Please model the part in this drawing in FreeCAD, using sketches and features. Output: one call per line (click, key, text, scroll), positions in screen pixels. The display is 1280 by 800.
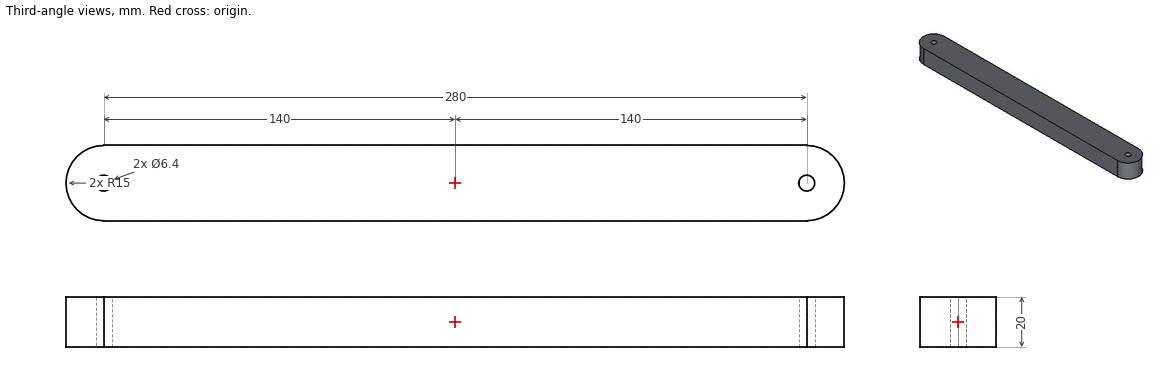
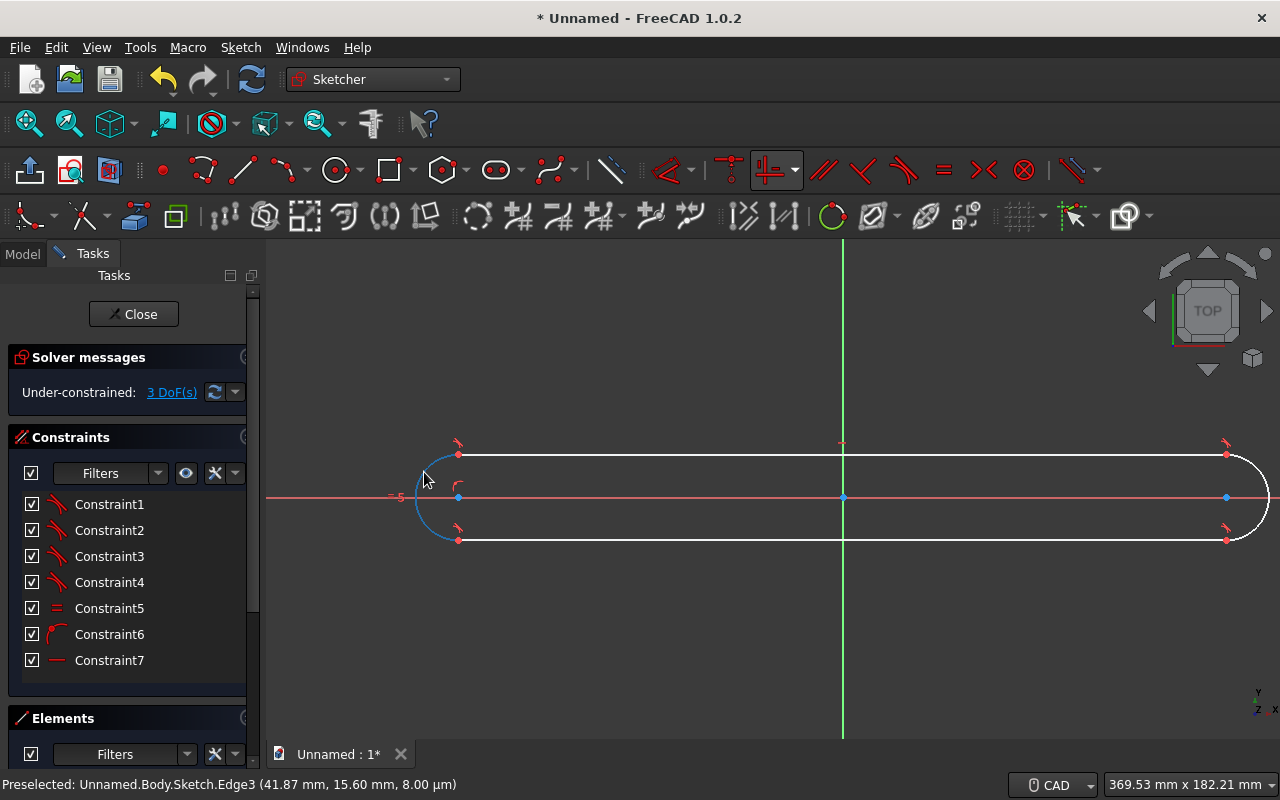
click(424, 472)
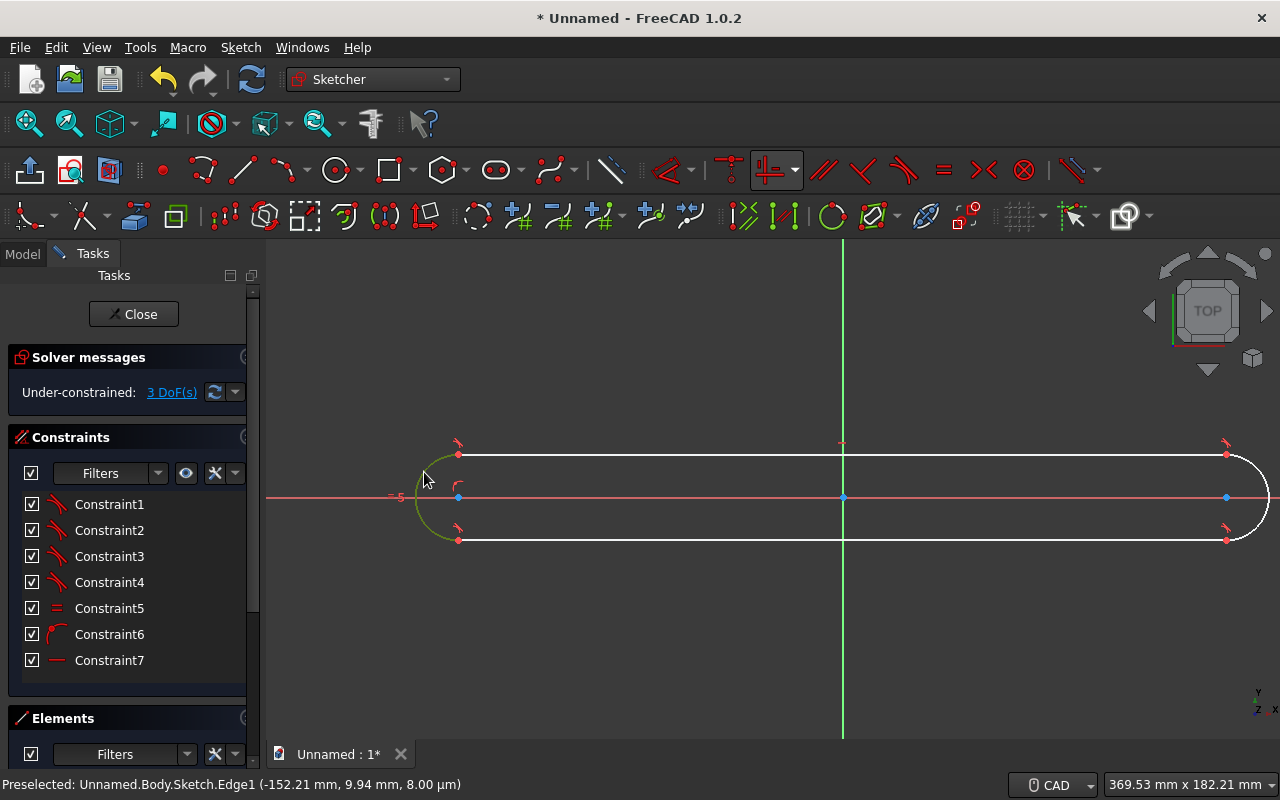
key(k)
key(r)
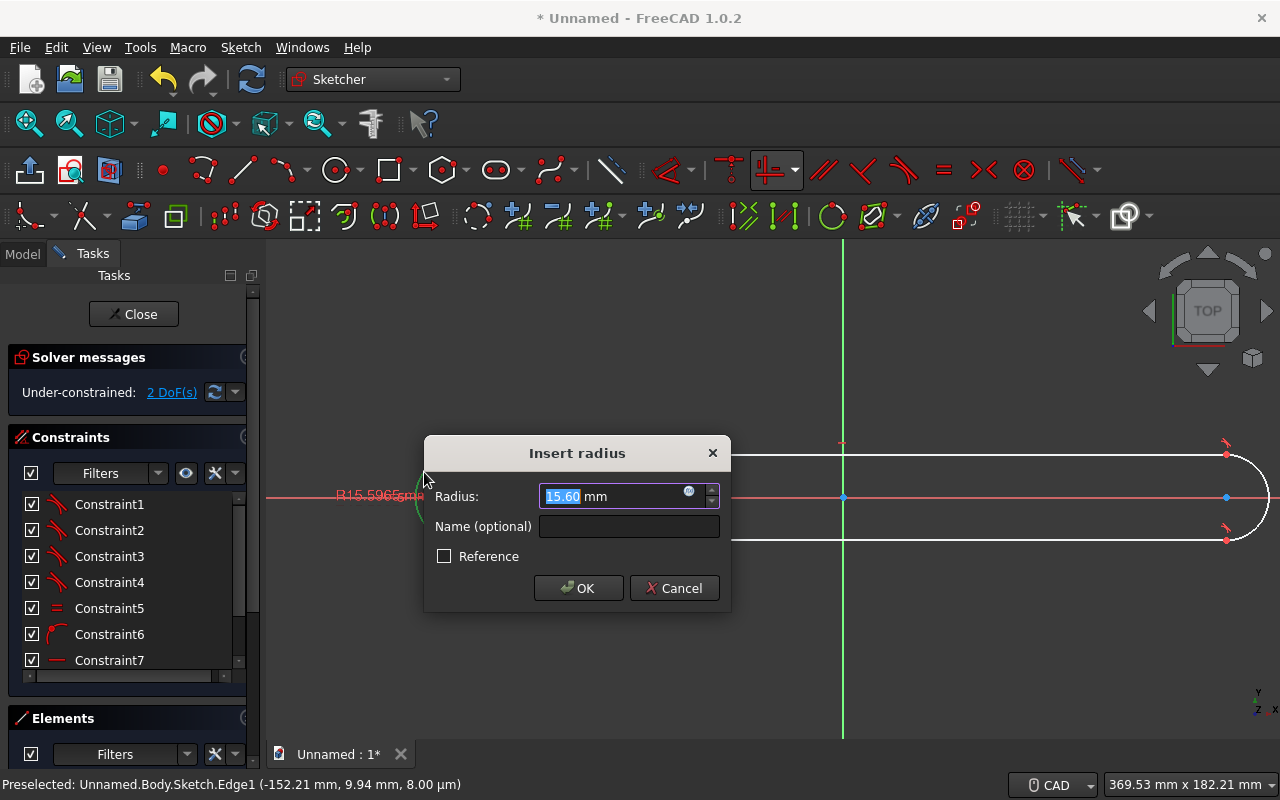
text(15)
key(Return)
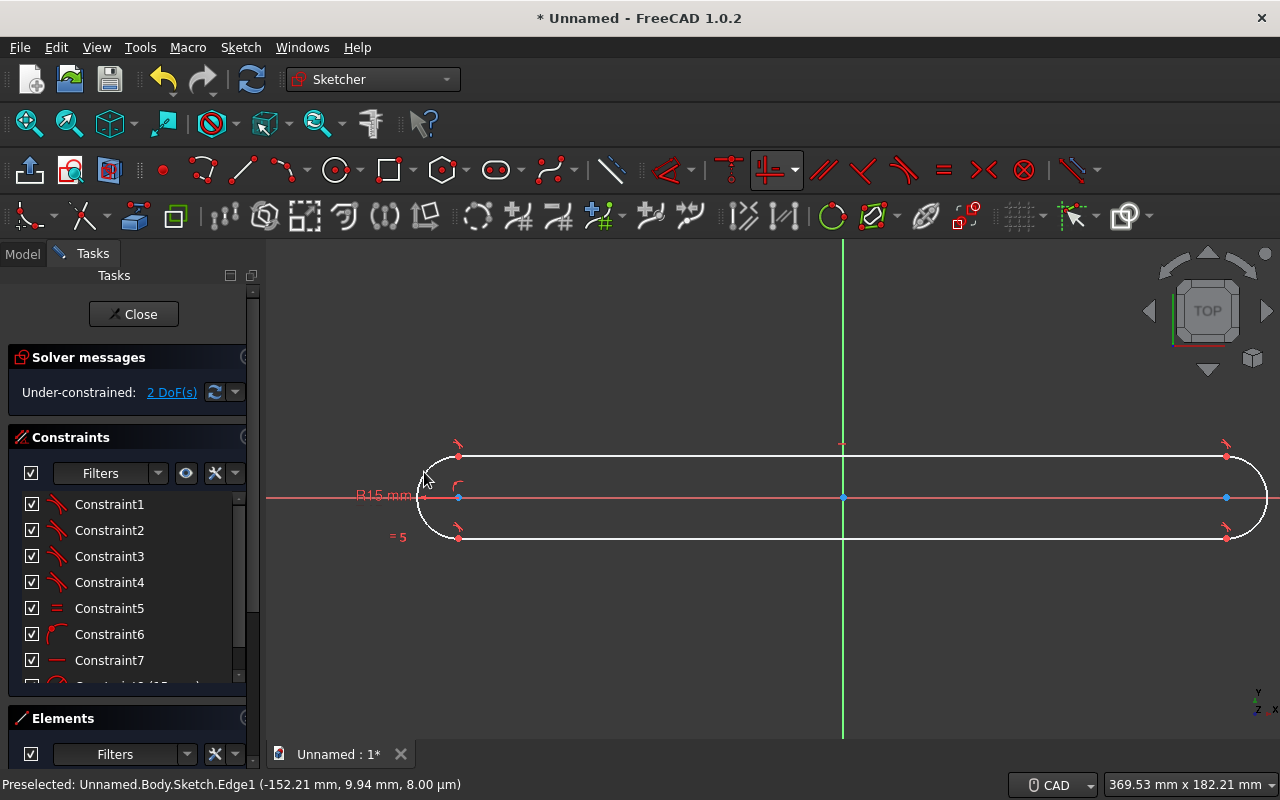
click(689, 456)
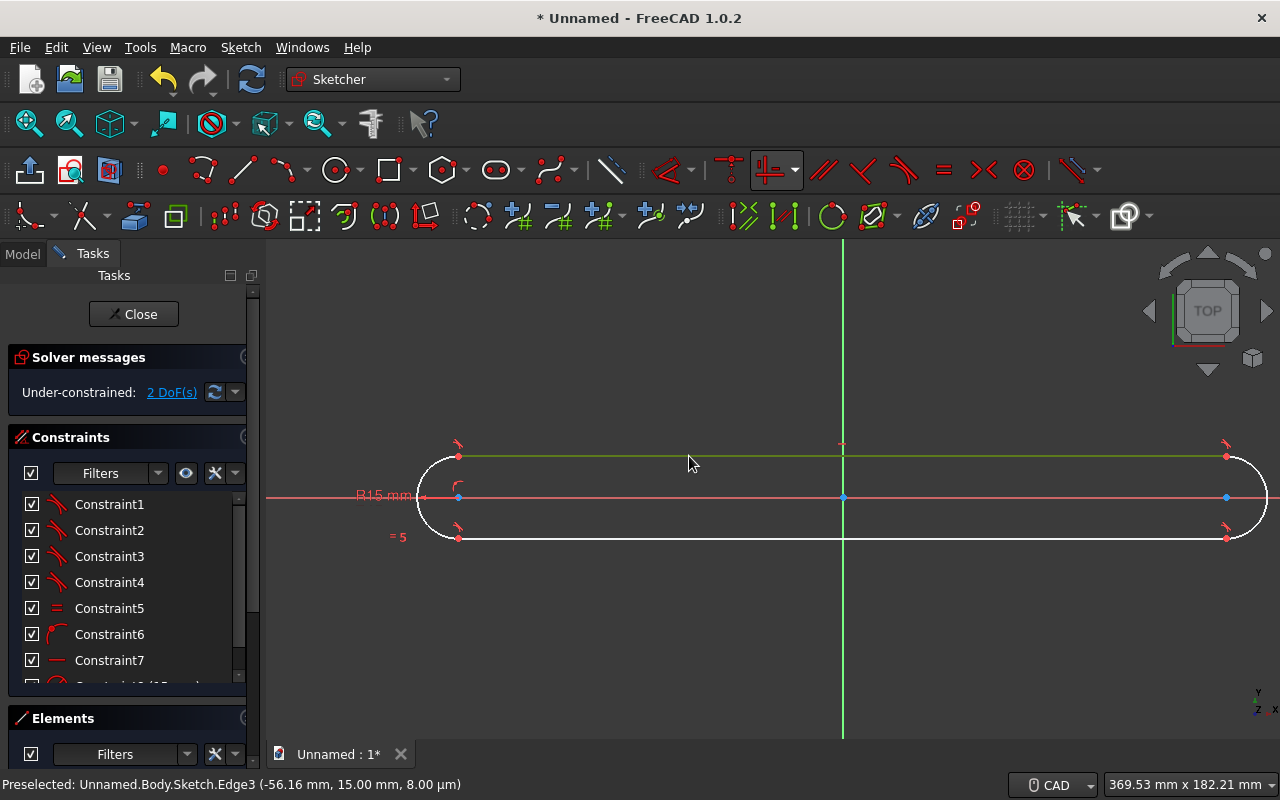
key(l)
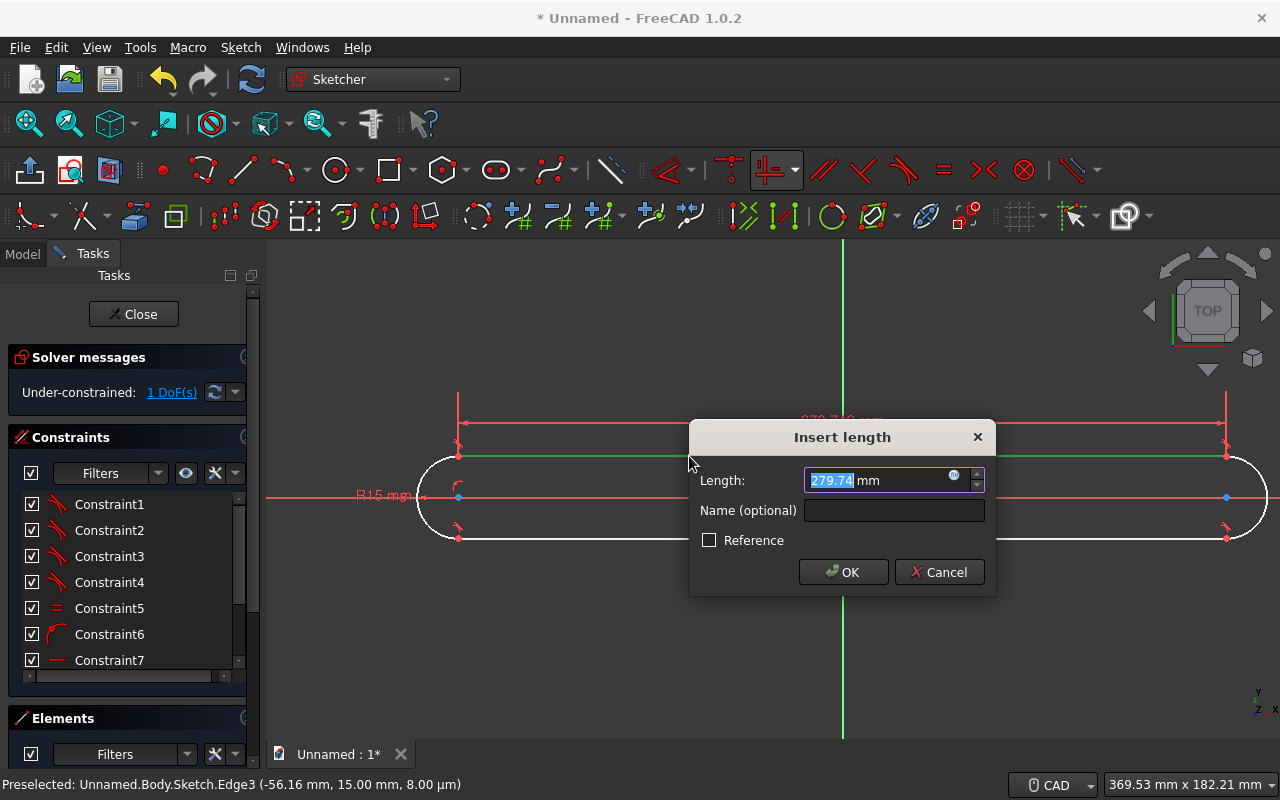
text(280)
key(Return)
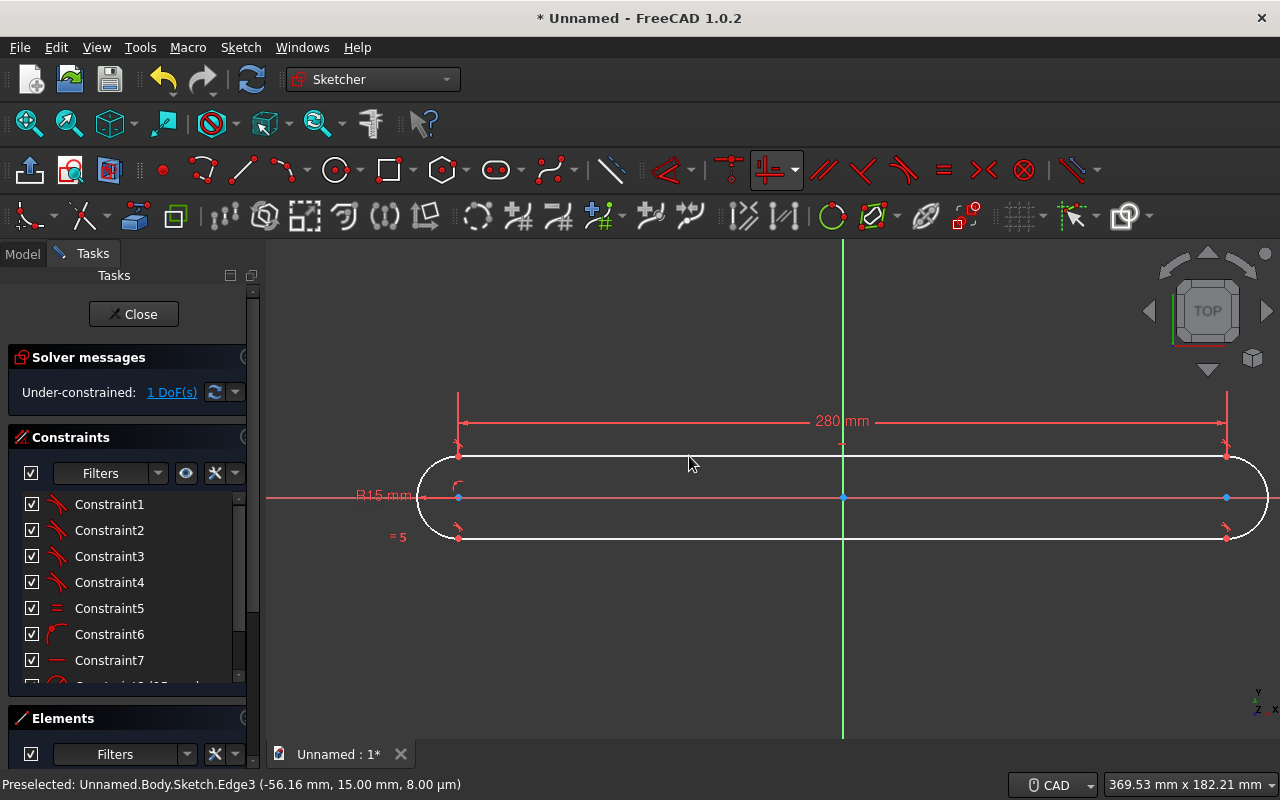
click(458, 456)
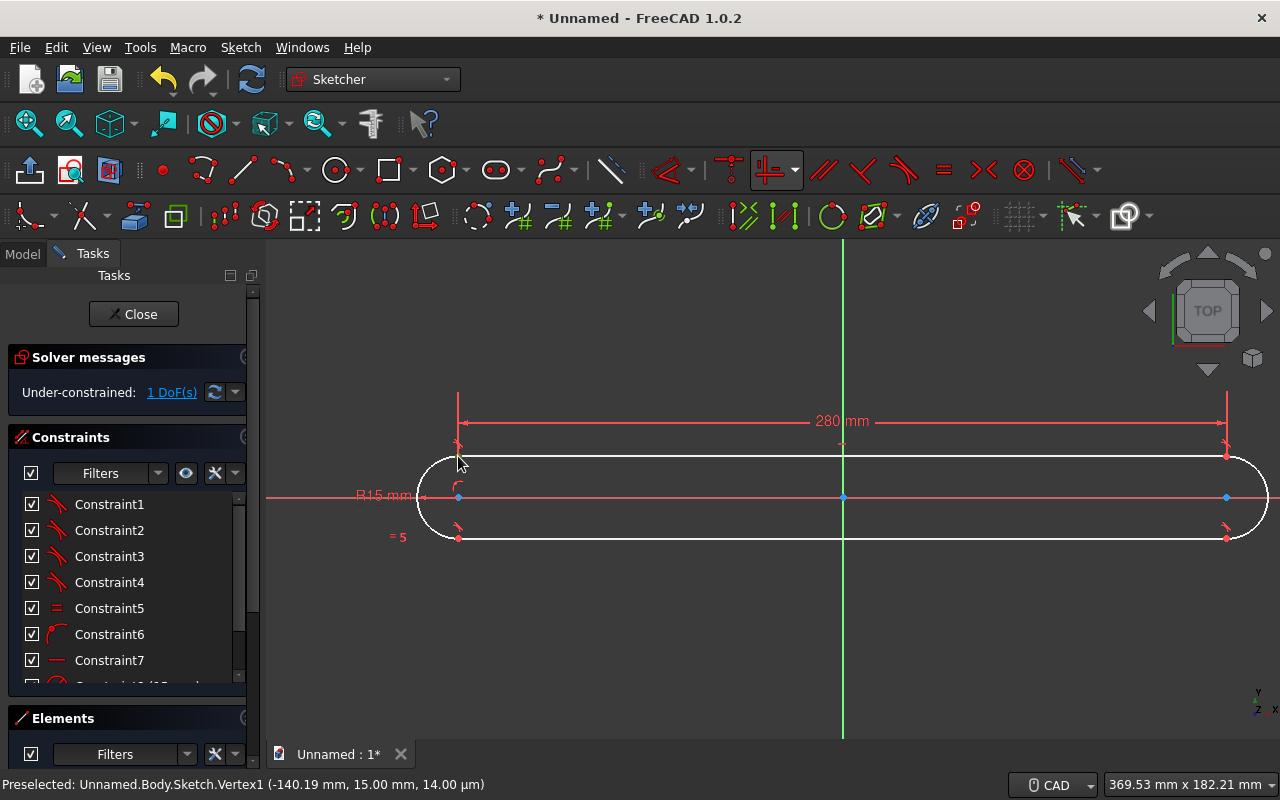
key(l)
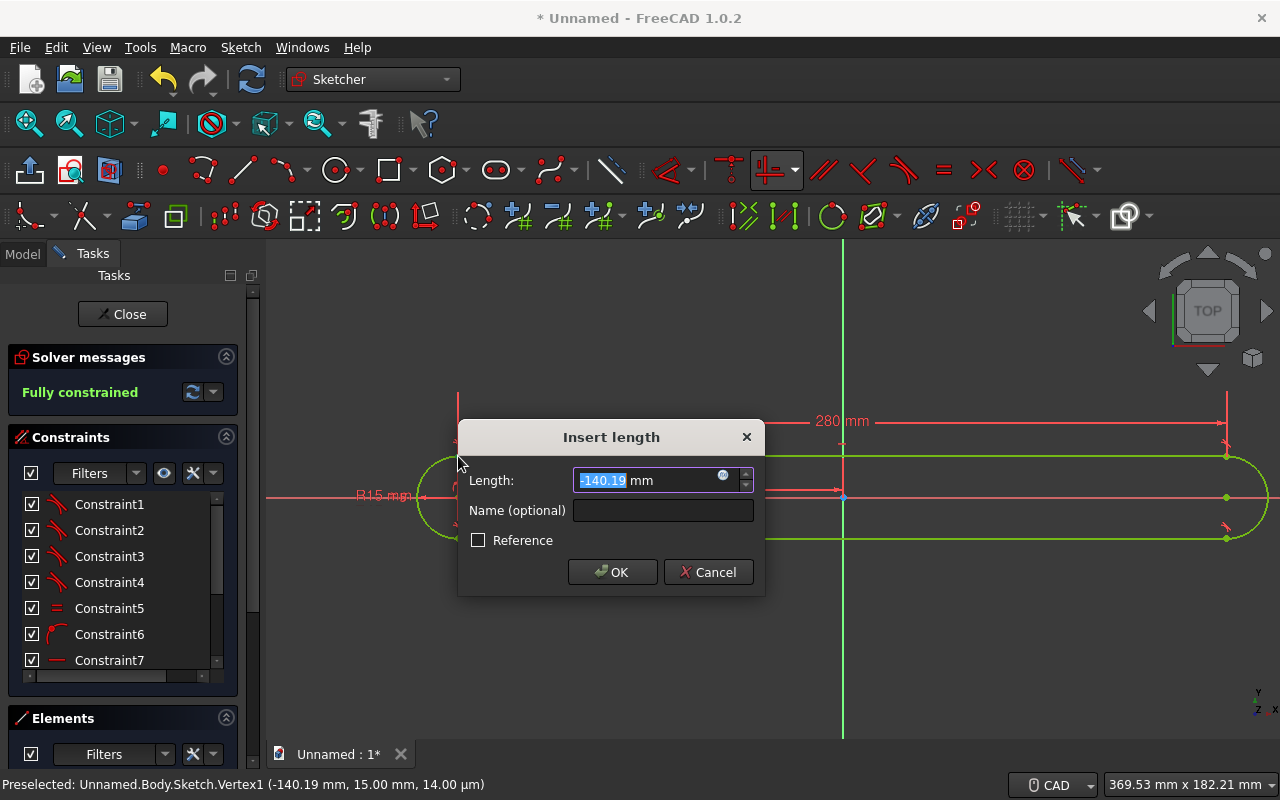
text(-140)
key(Return)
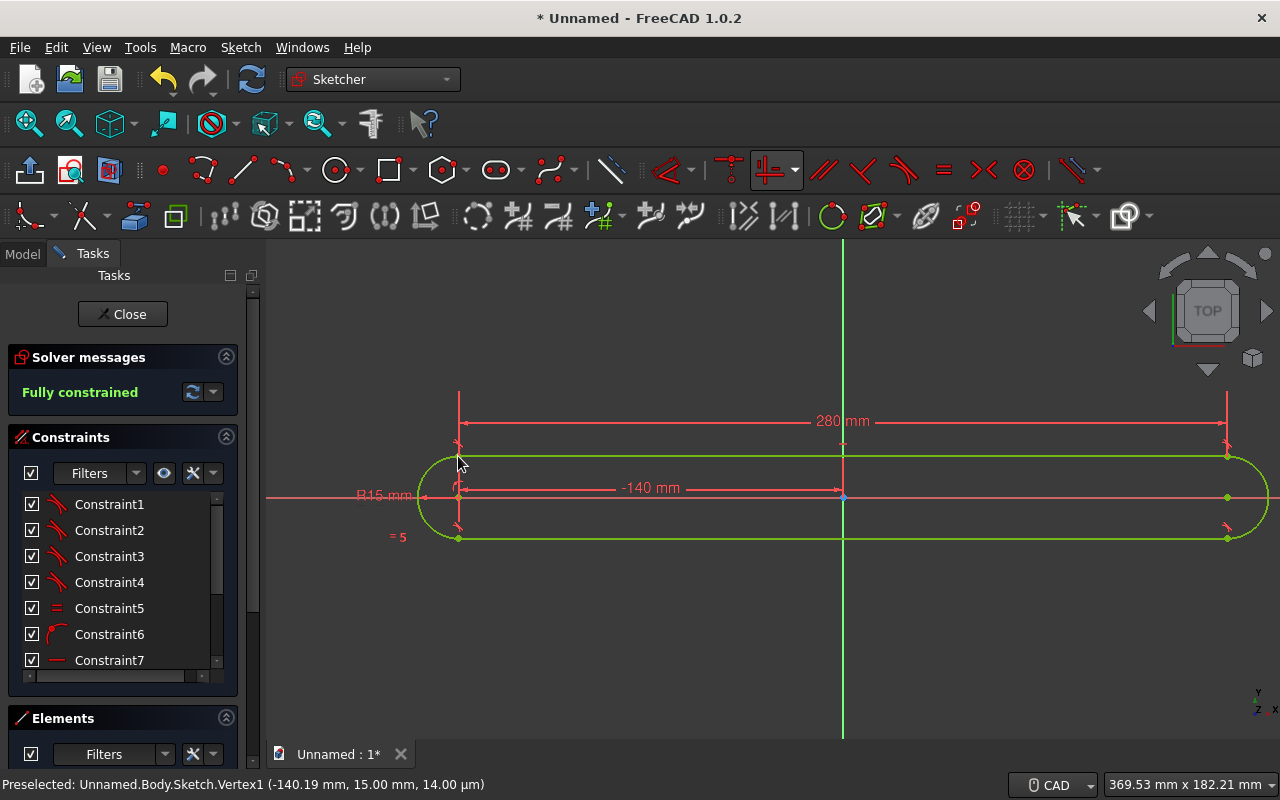
click(123, 314)